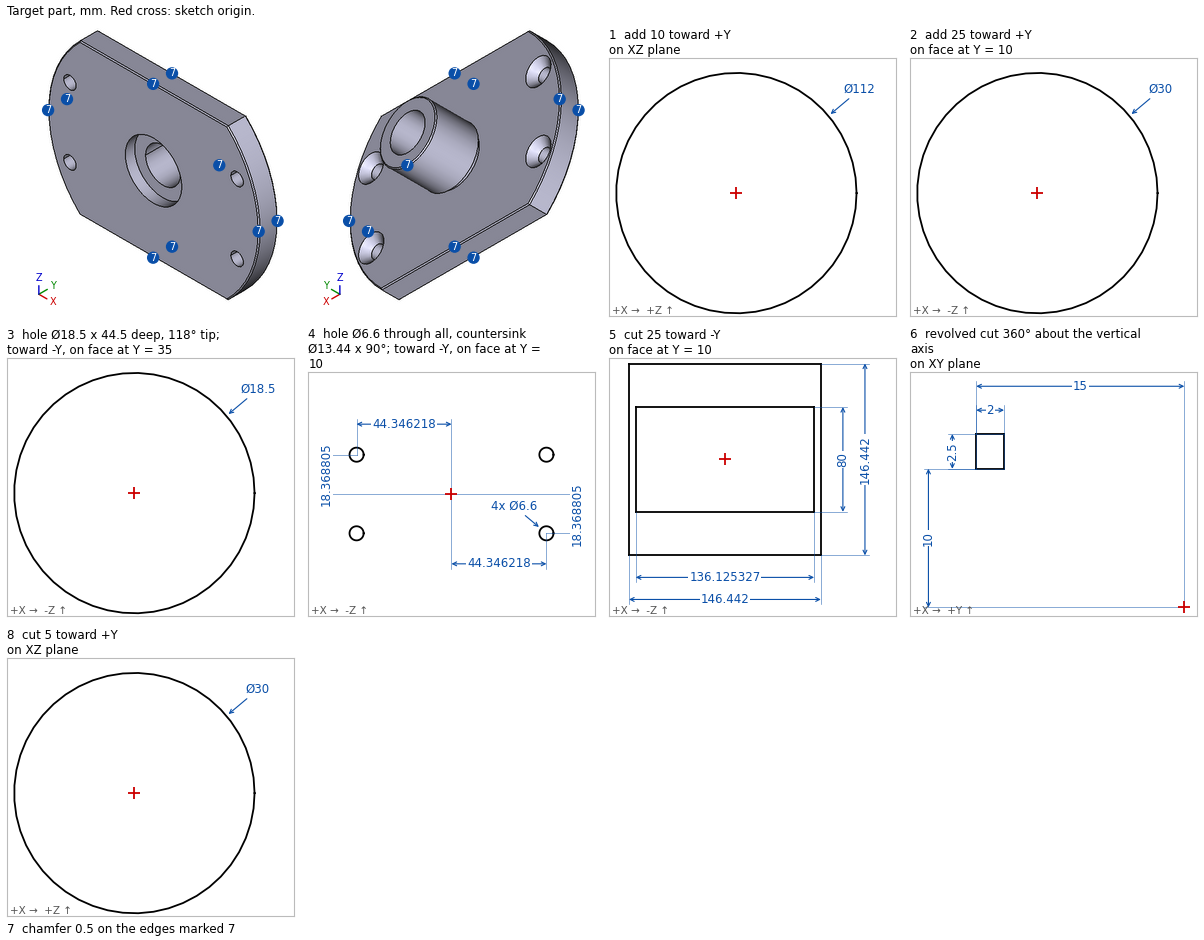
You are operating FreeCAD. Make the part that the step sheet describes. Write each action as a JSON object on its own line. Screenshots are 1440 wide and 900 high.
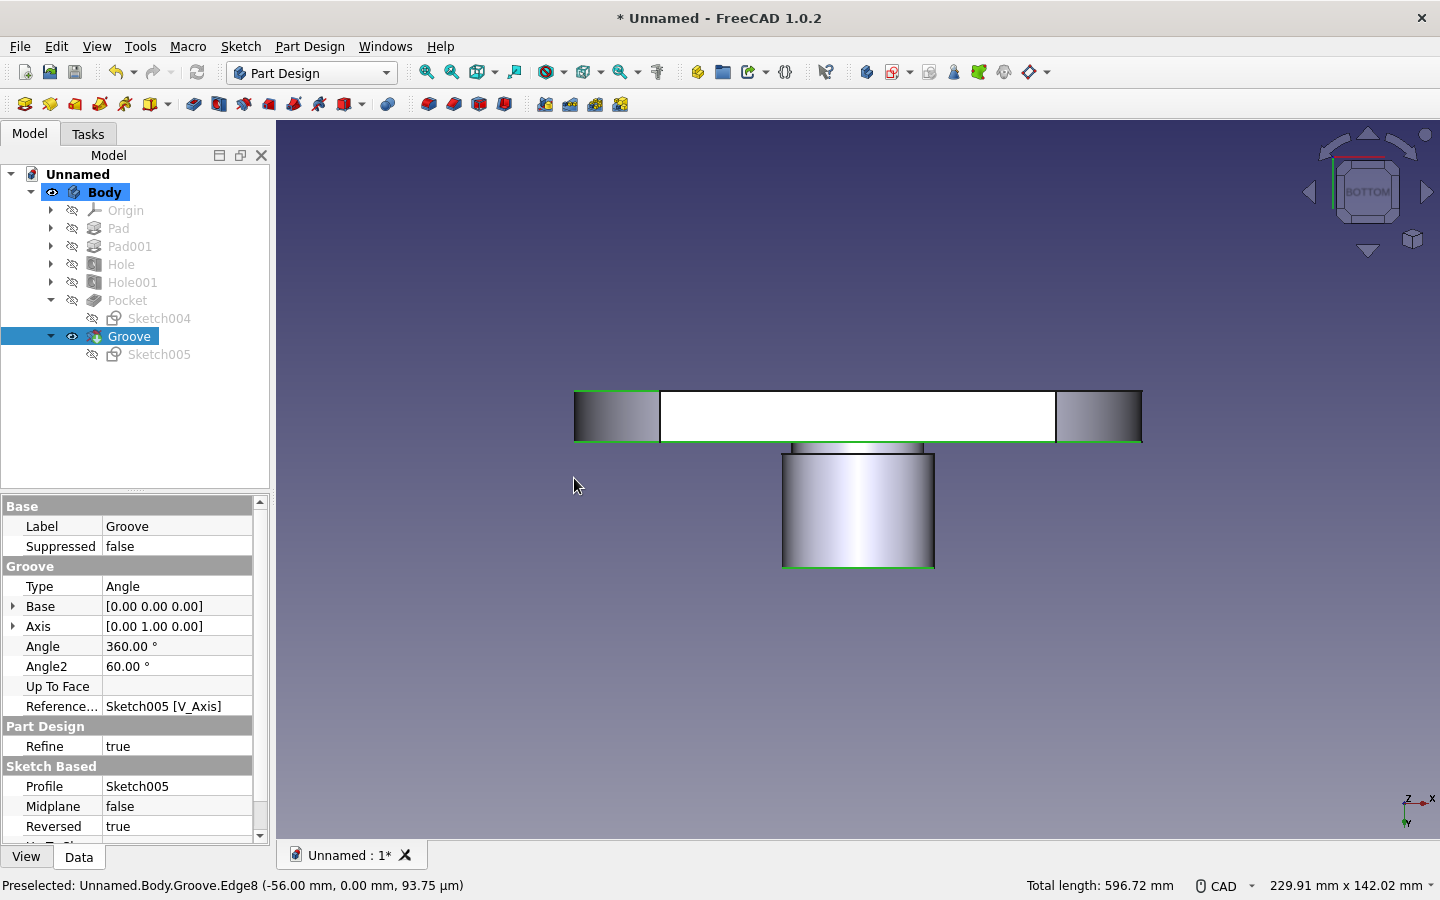
{"action": "left_click", "coordinate": [858, 390], "text": "ctrl"}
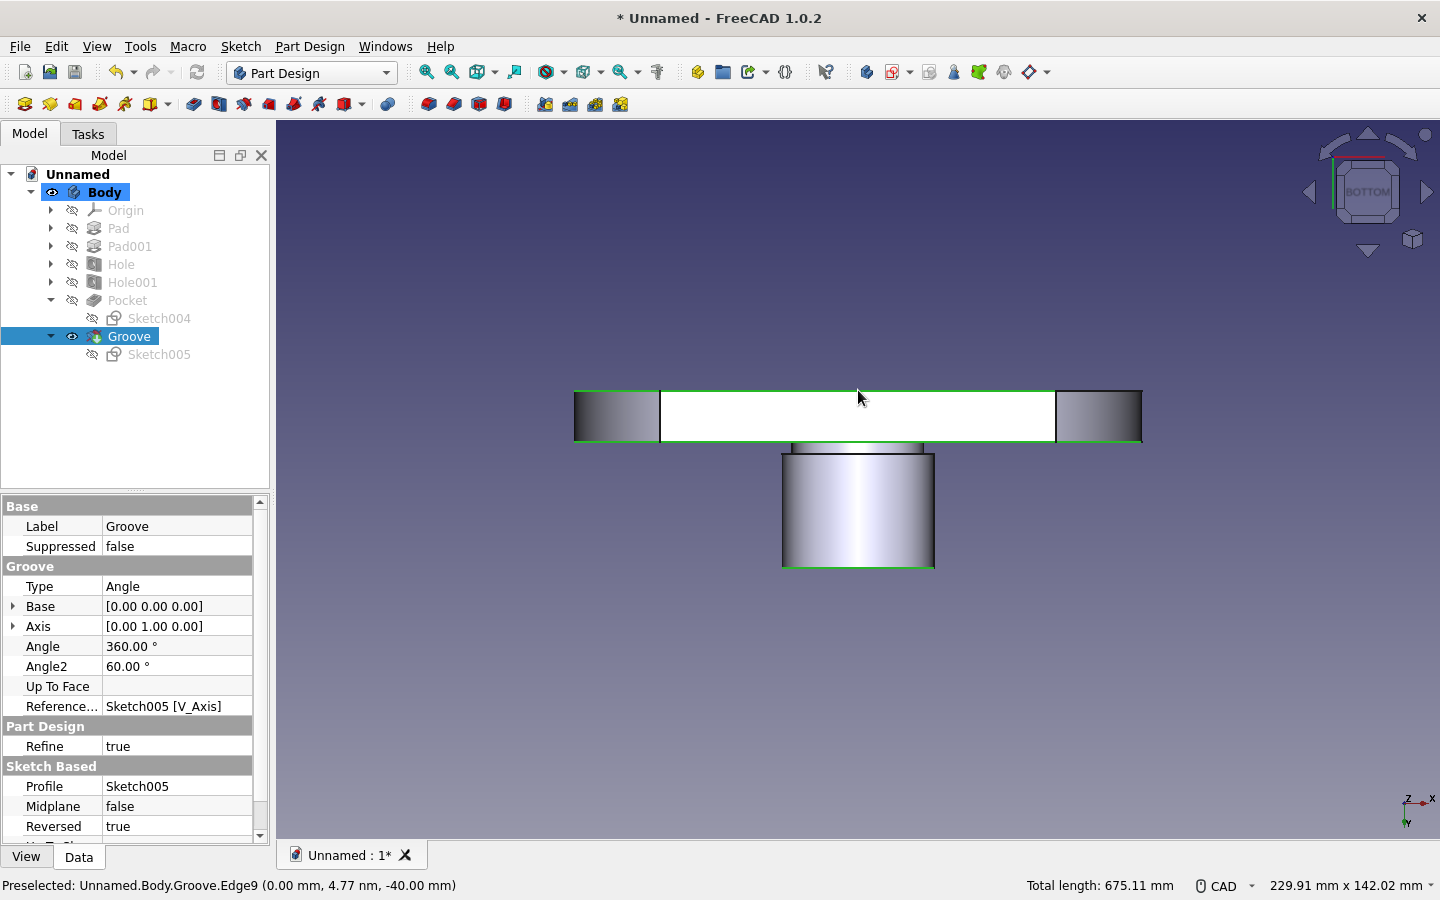
{"action": "left_click", "coordinate": [454, 104]}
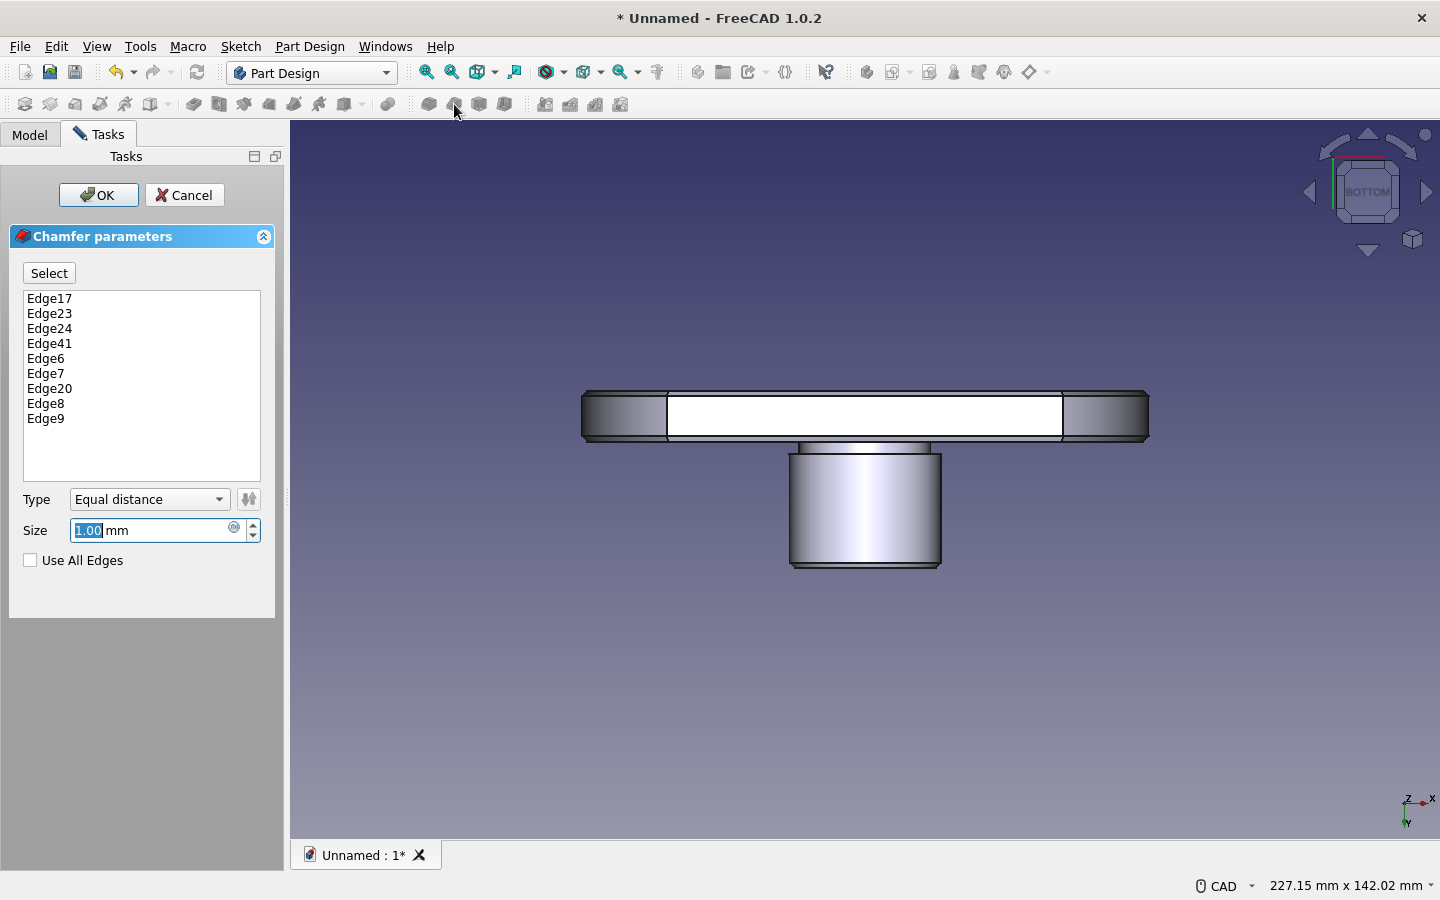
{"action": "type", "text": "0.5"}
{"action": "key", "text": "Tab"}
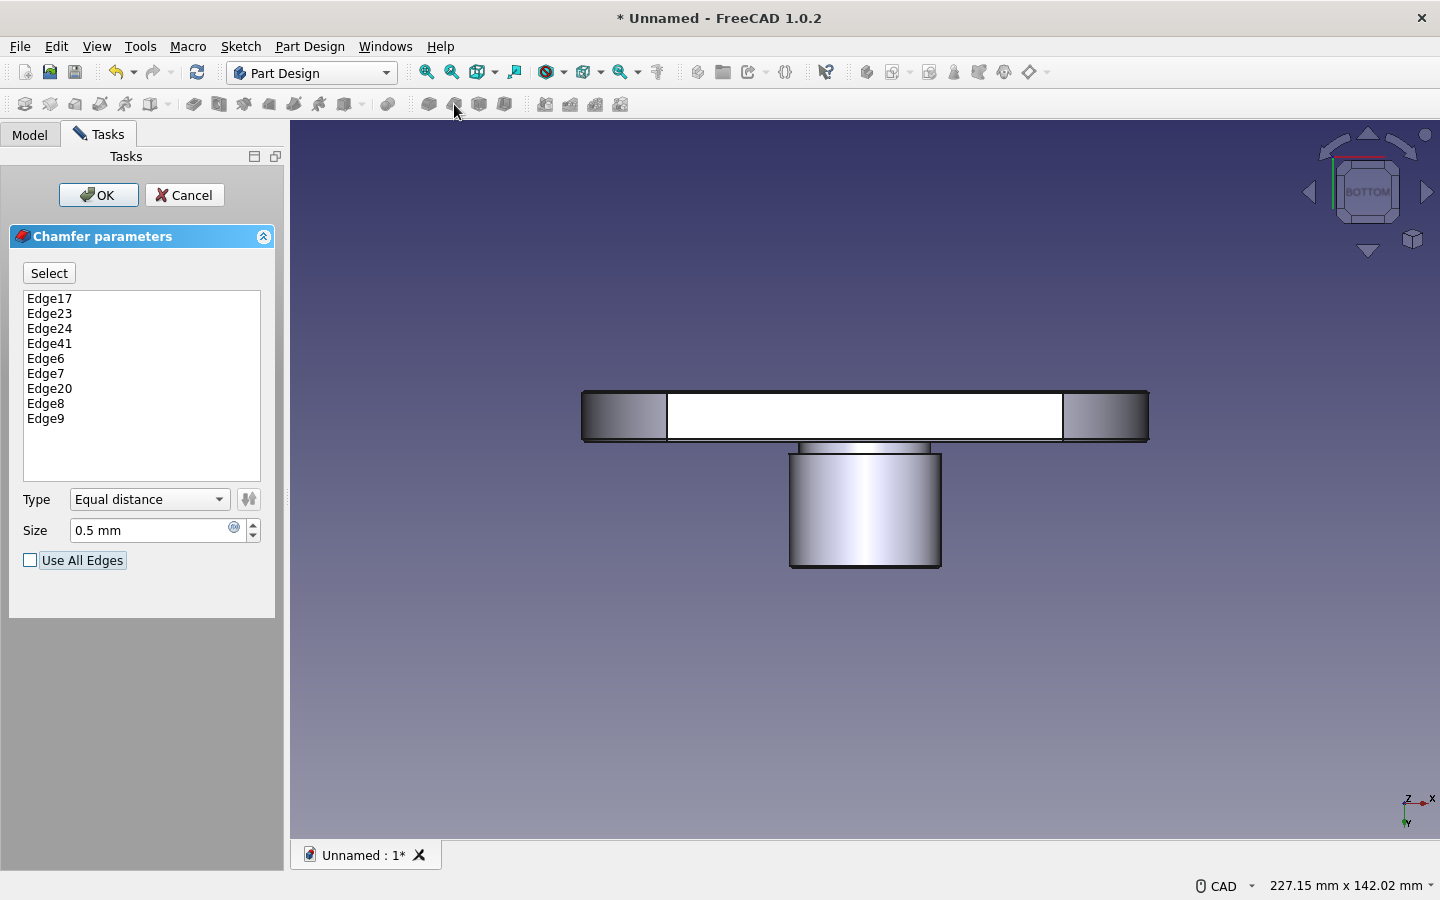
{"action": "left_click", "coordinate": [99, 195]}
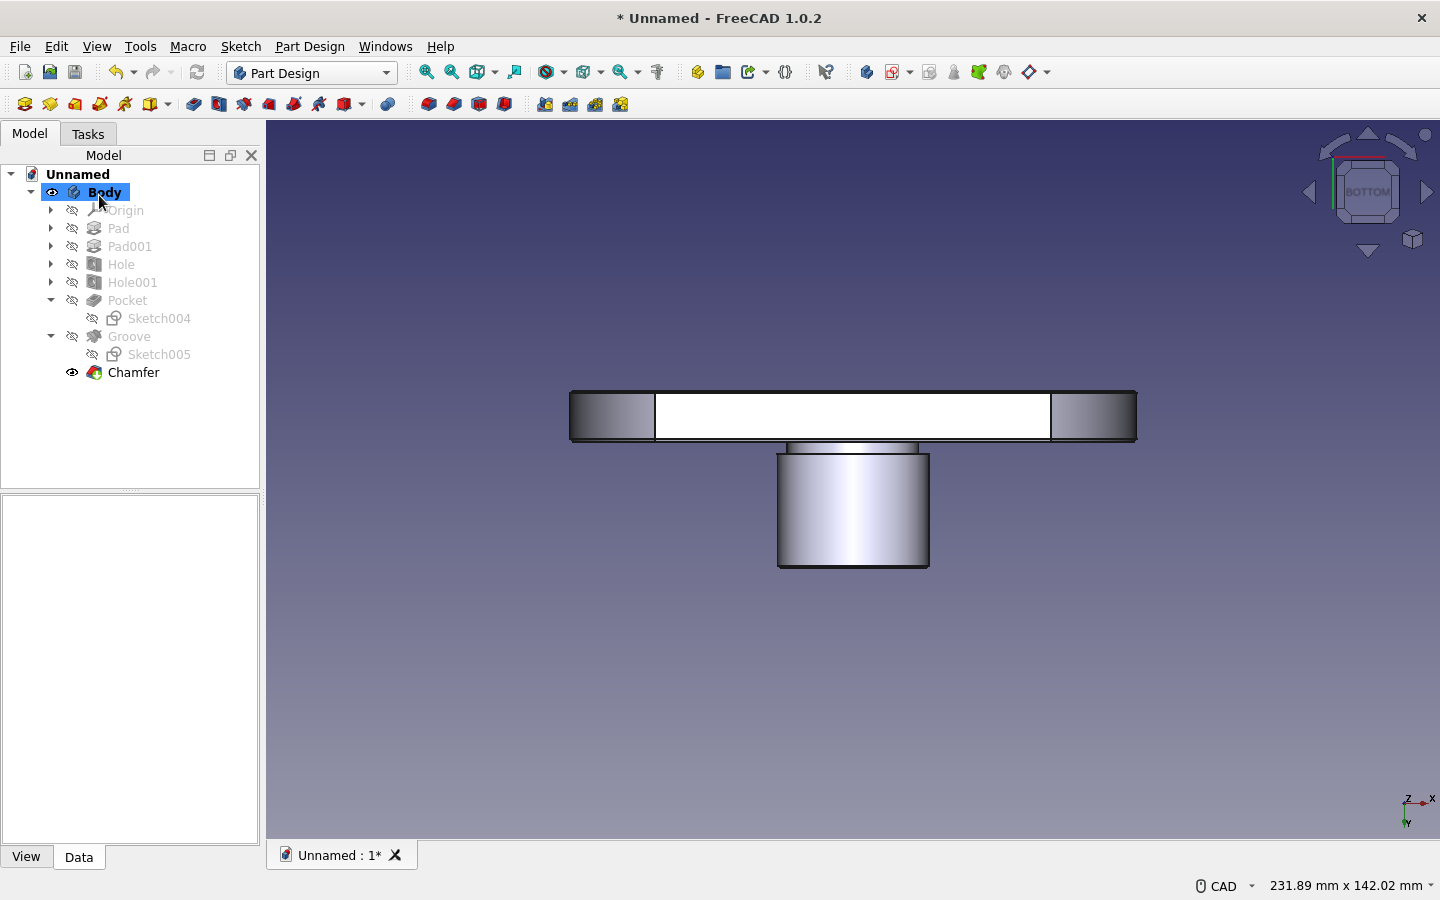
{"action": "left_click", "coordinate": [892, 72]}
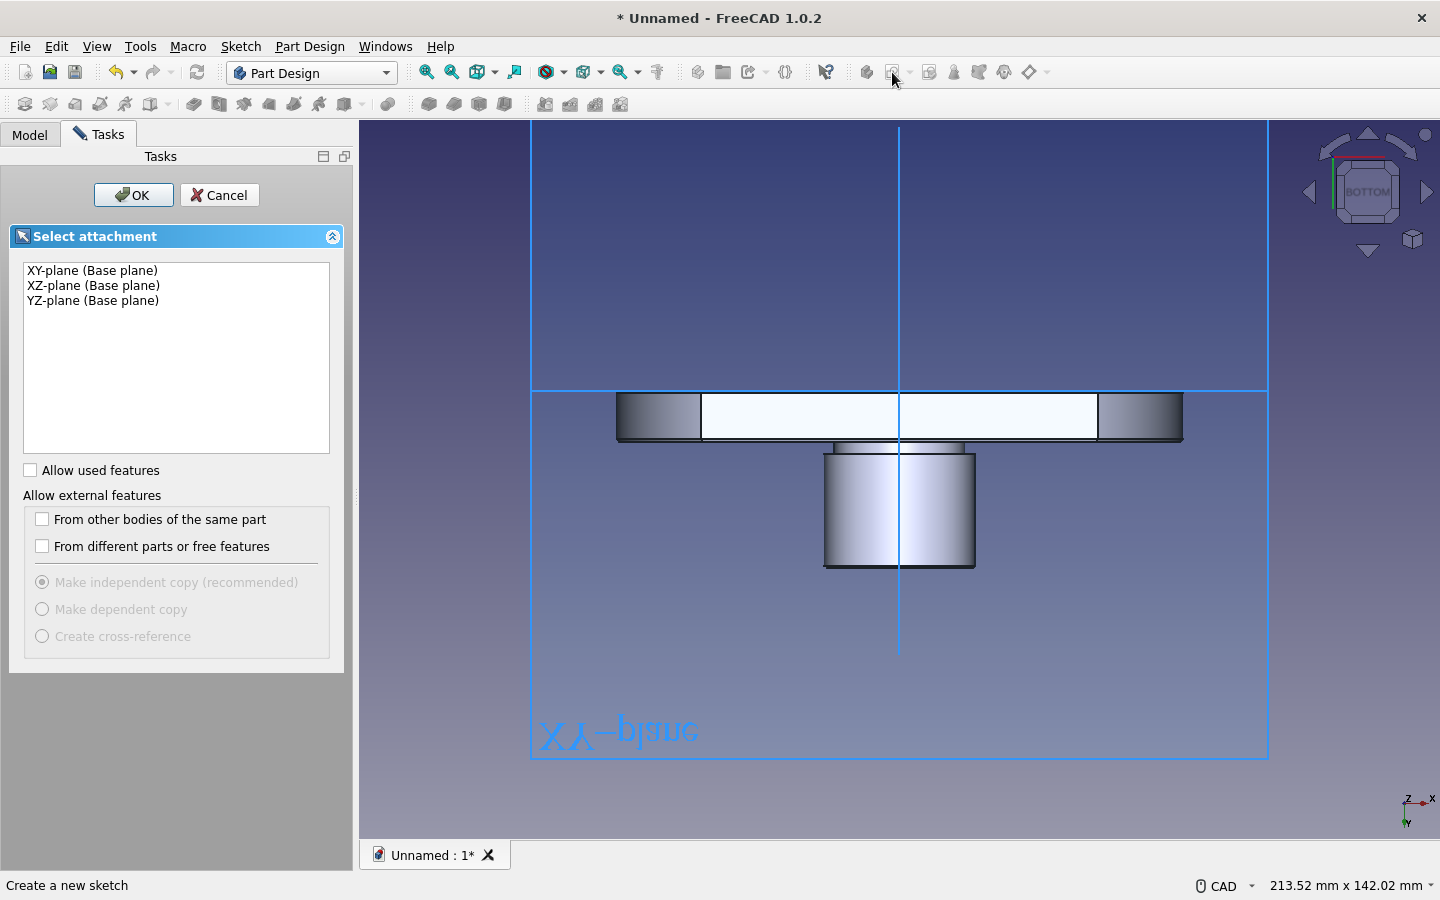
{"action": "left_click", "coordinate": [84, 286]}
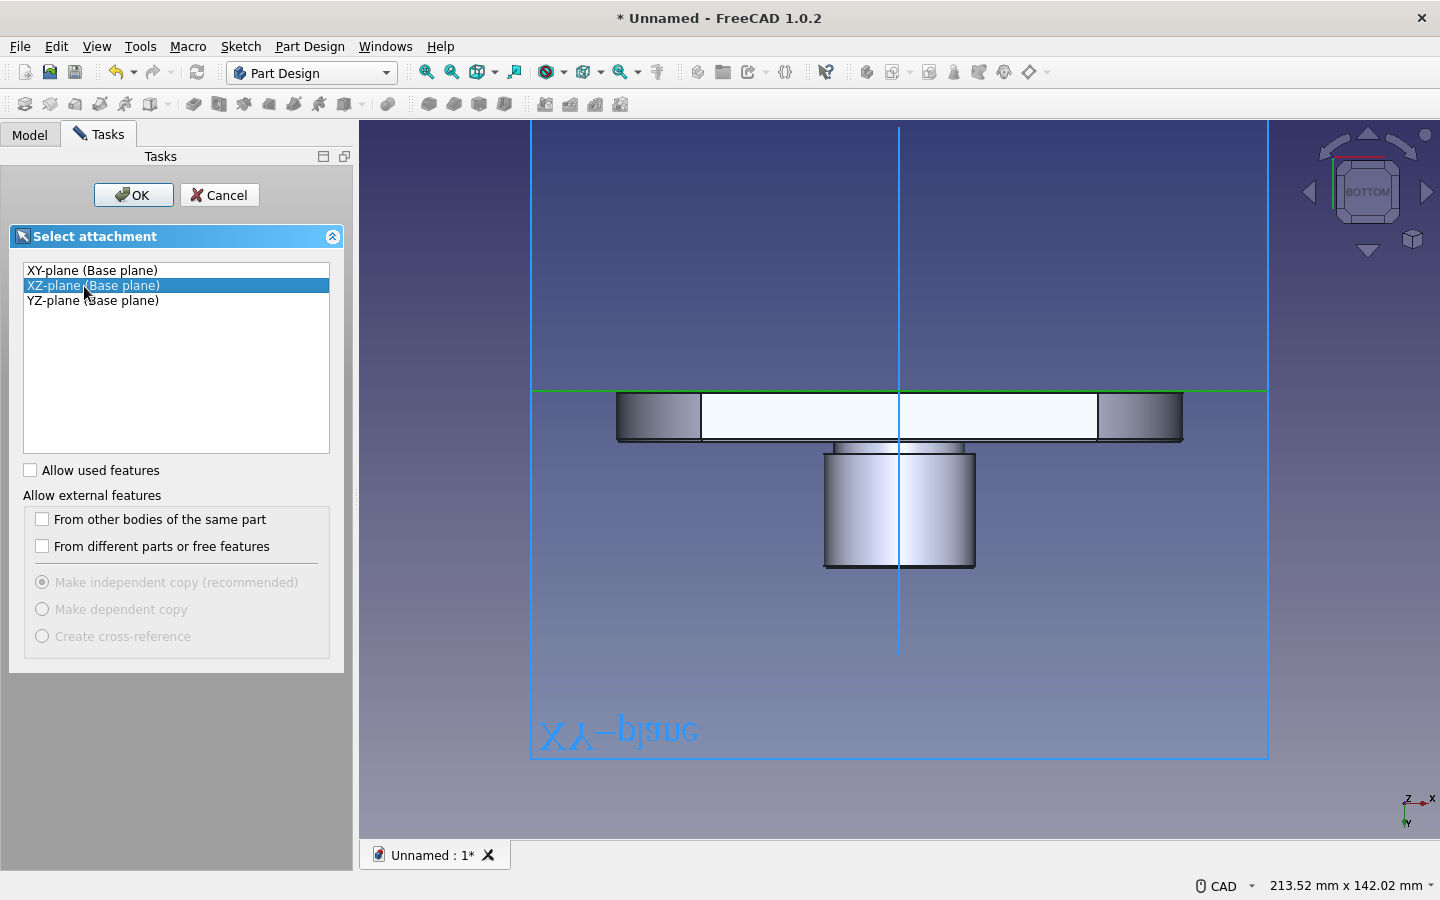
{"action": "left_click", "coordinate": [134, 195]}